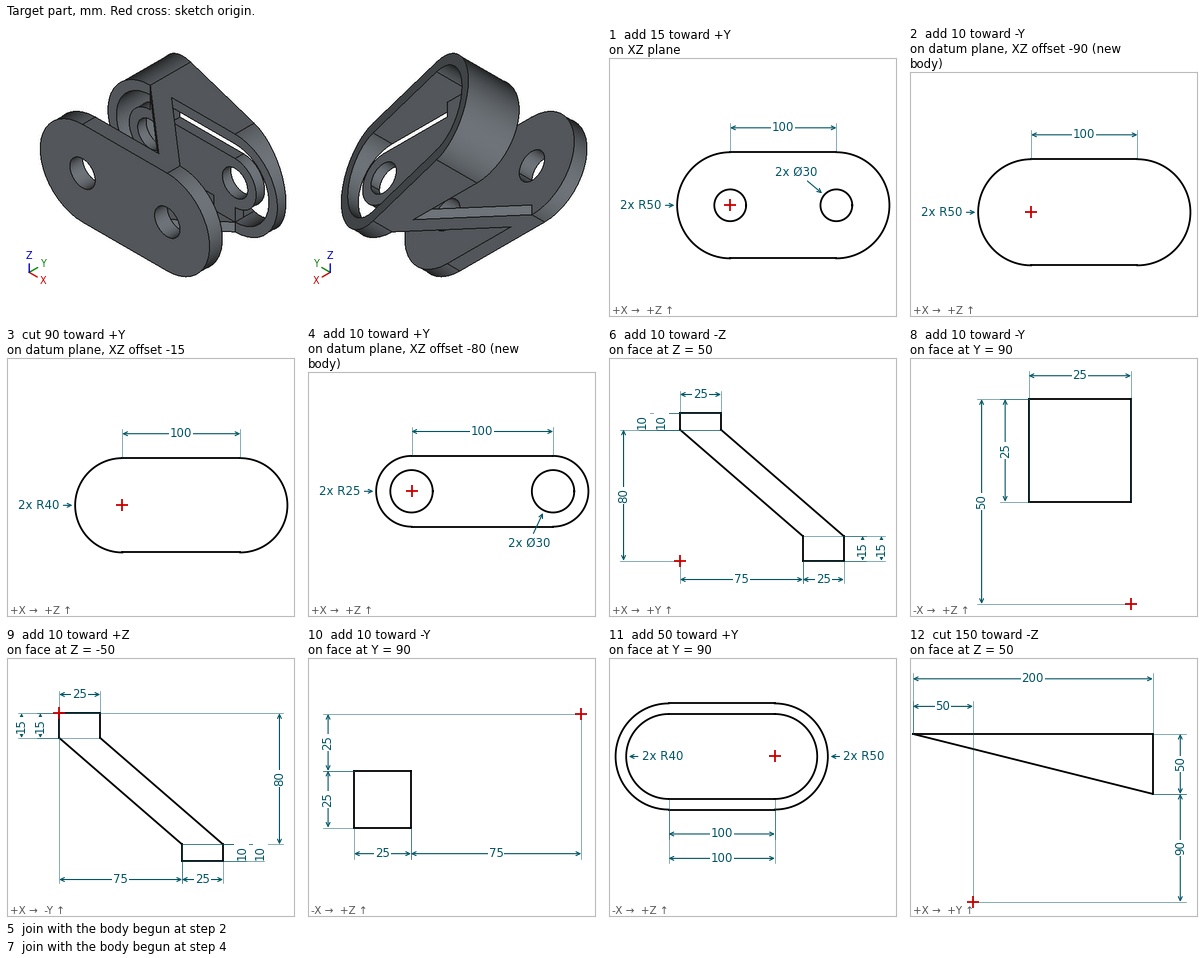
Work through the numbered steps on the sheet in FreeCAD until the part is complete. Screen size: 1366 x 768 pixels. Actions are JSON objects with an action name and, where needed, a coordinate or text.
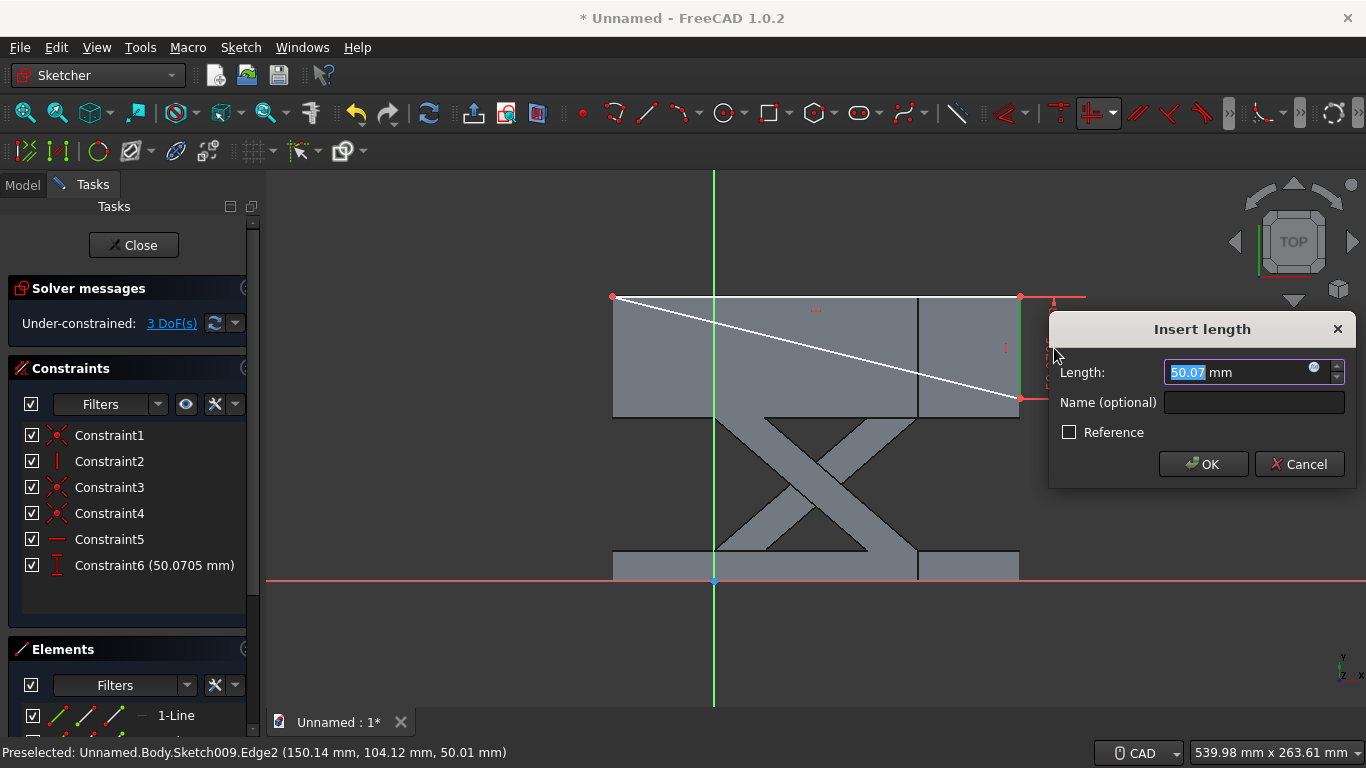
{"action": "type", "text": "50"}
{"action": "key", "text": "Return"}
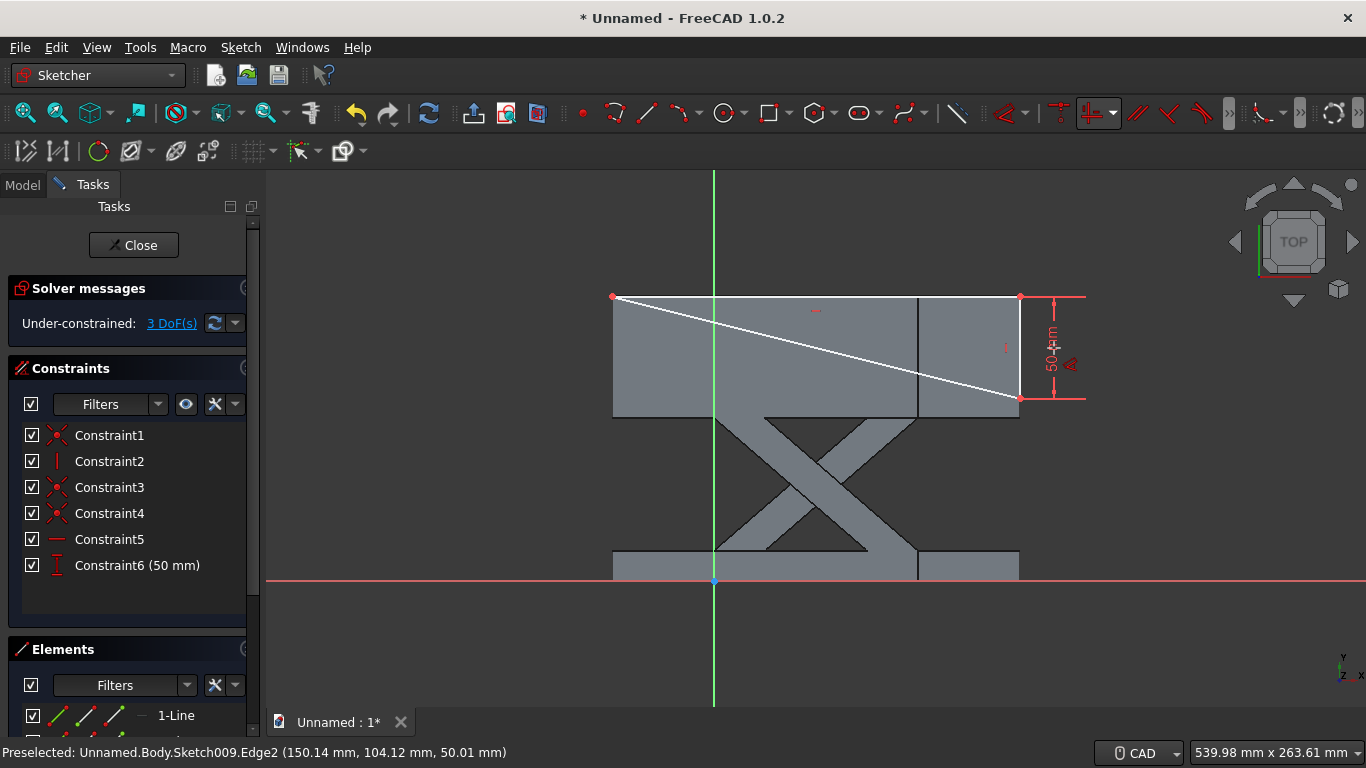
{"action": "left_click", "coordinate": [898, 297]}
{"action": "left_click", "coordinate": [816, 263]}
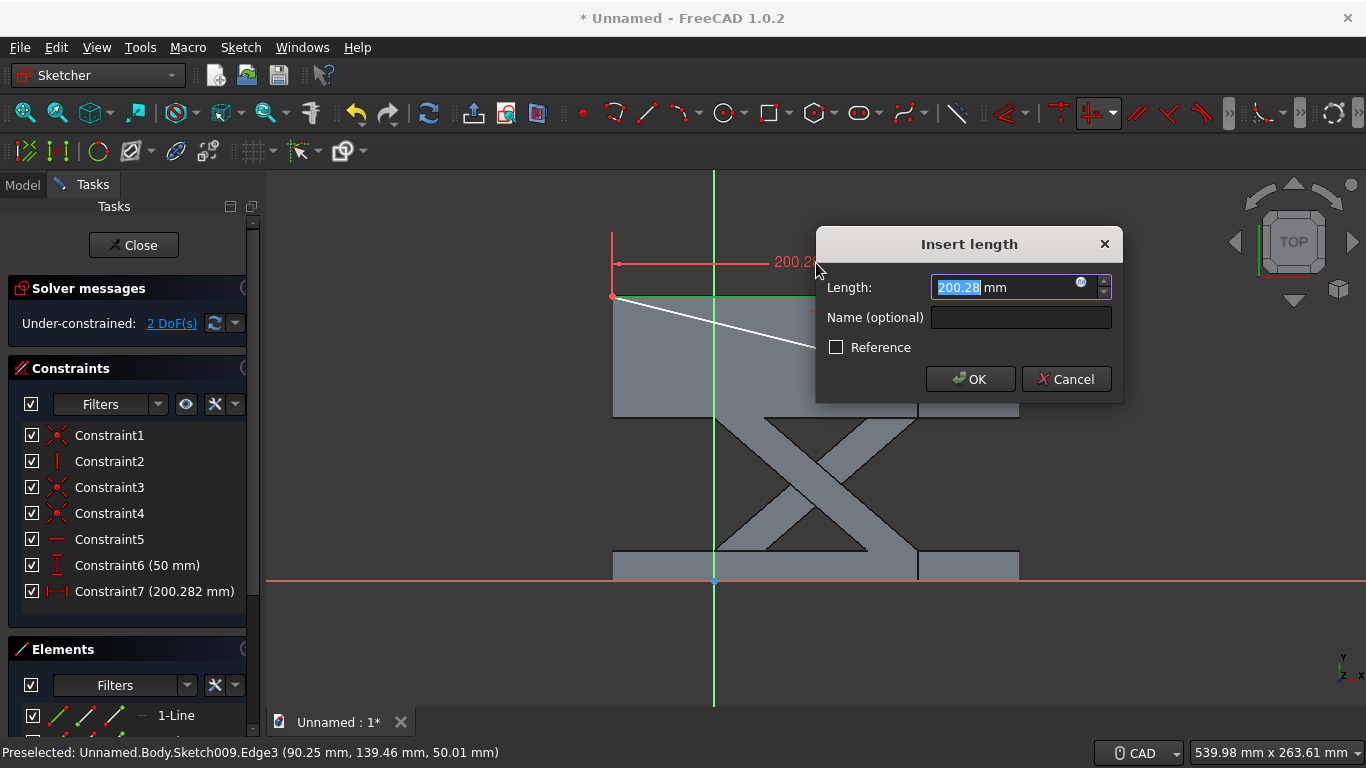
{"action": "type", "text": "200"}
{"action": "key", "text": "Return"}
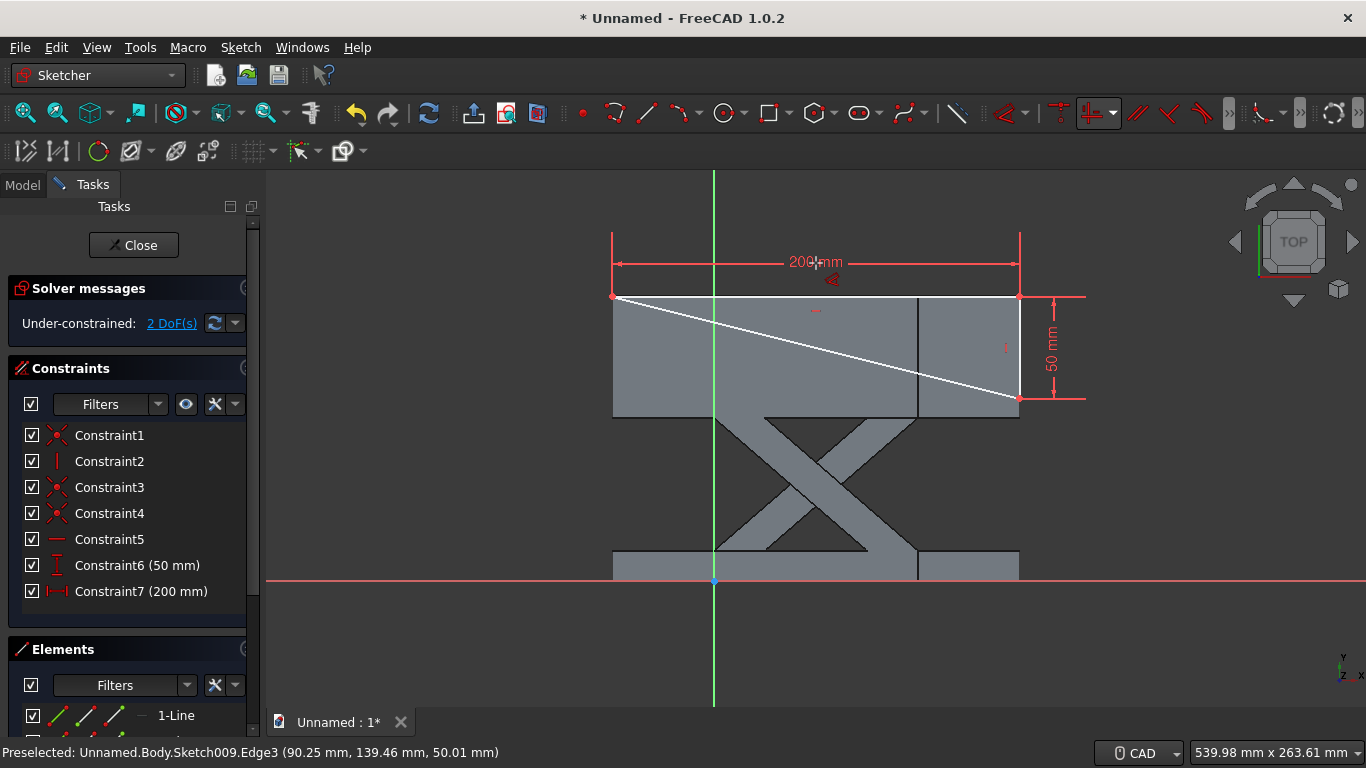
{"action": "left_click", "coordinate": [612, 297]}
{"action": "left_click", "coordinate": [663, 615]}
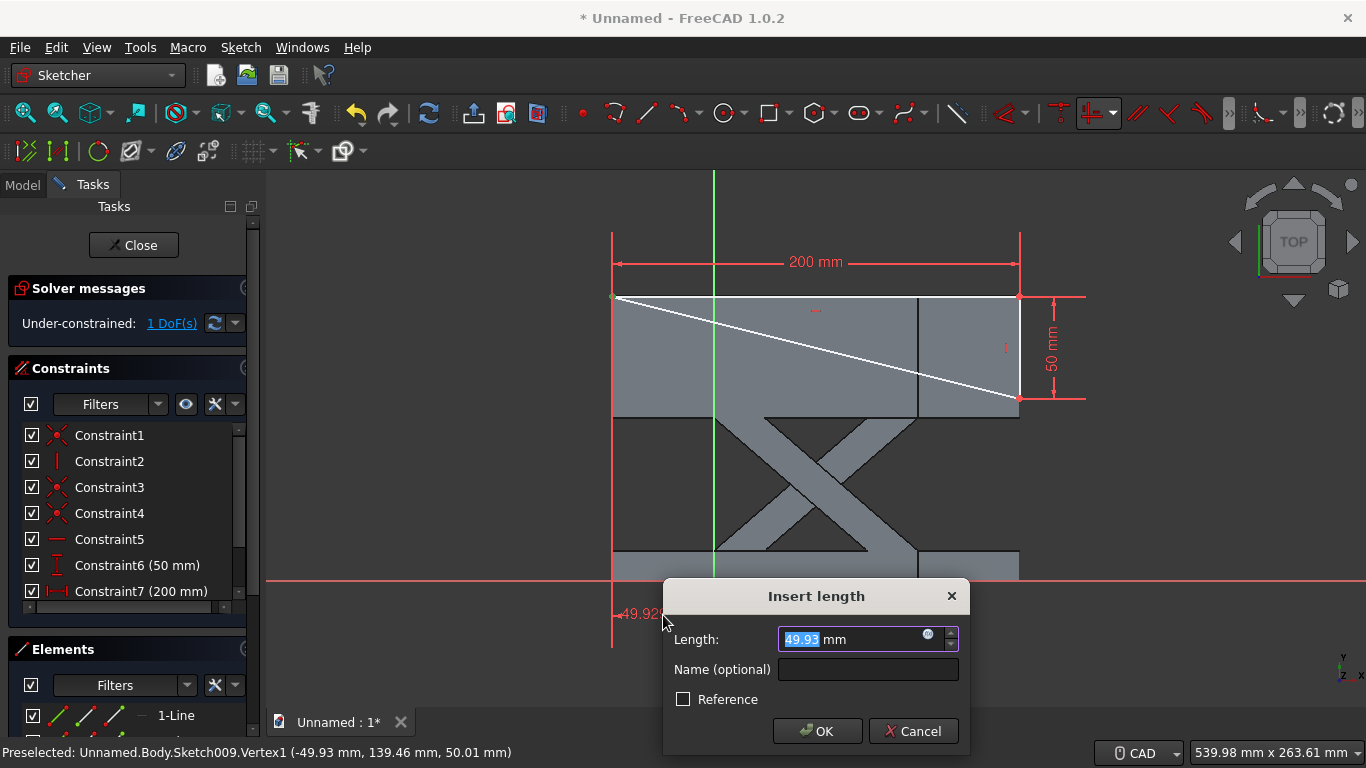
{"action": "type", "text": "50"}
{"action": "key", "text": "Return"}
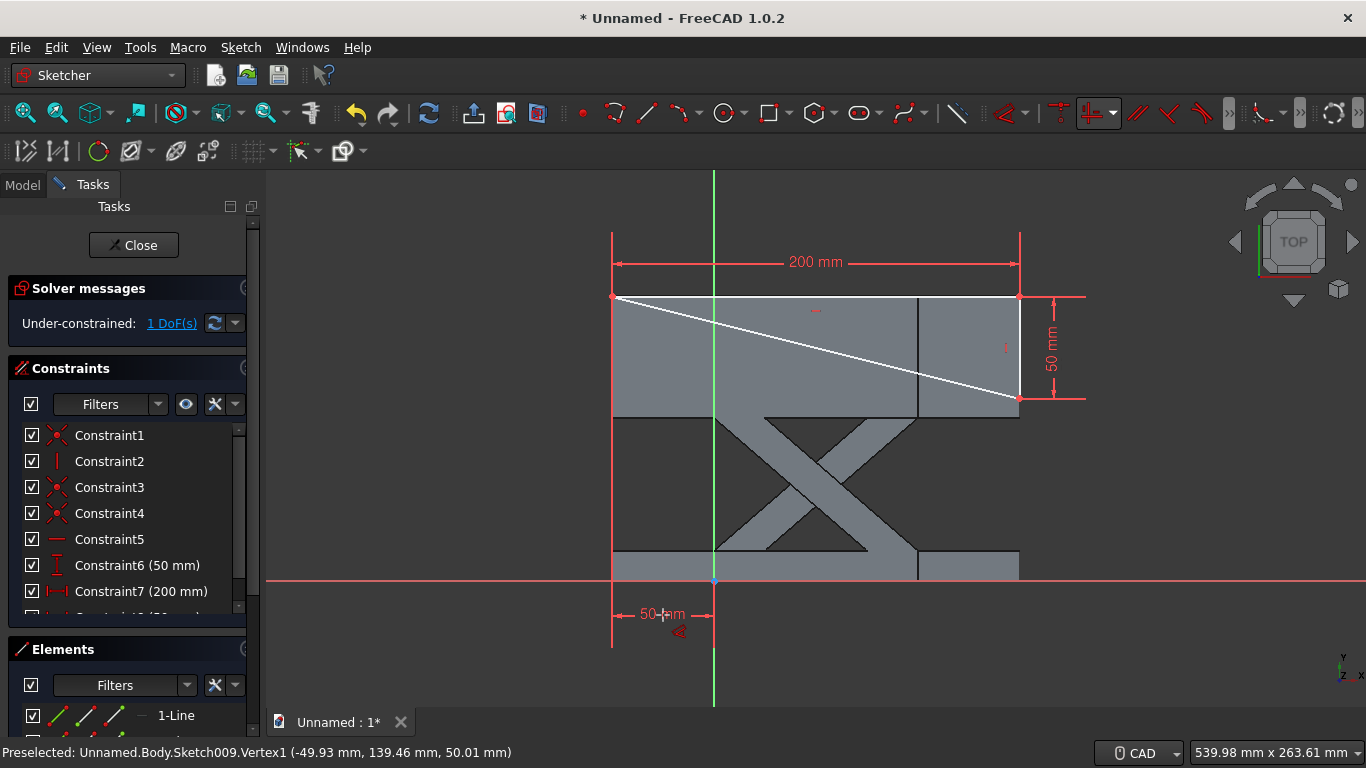
{"action": "left_click", "coordinate": [1020, 399]}
{"action": "left_click", "coordinate": [1054, 490]}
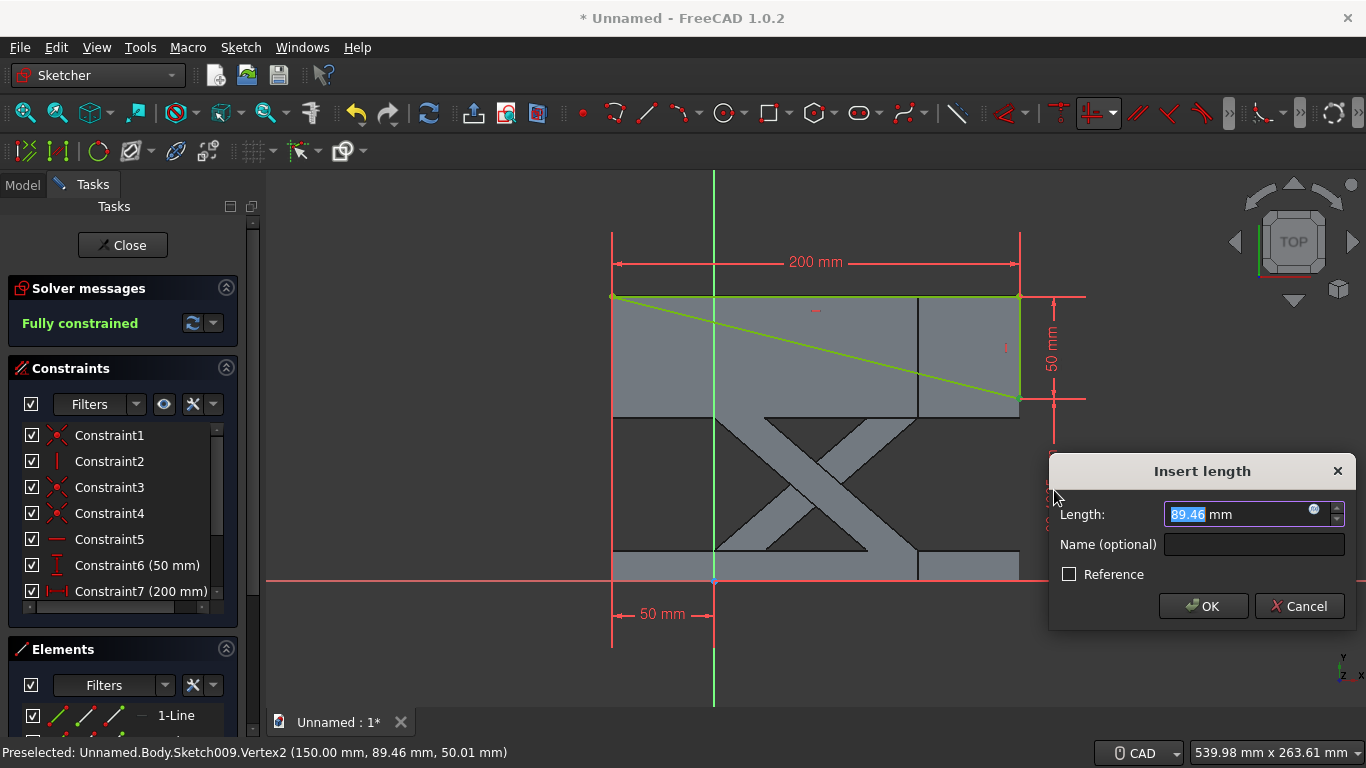
{"action": "type", "text": "90"}
{"action": "key", "text": "Return"}
{"action": "key", "text": "Escape"}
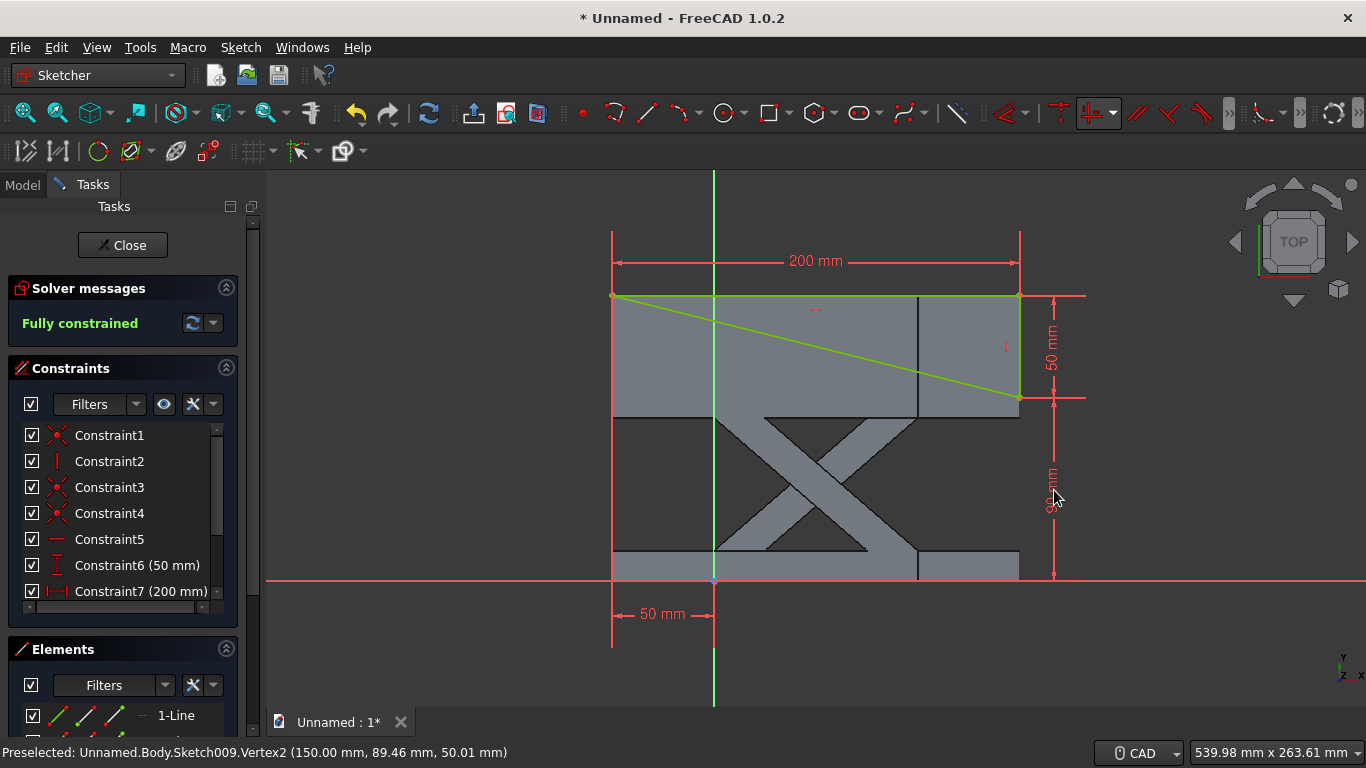
{"action": "left_click", "coordinate": [123, 245]}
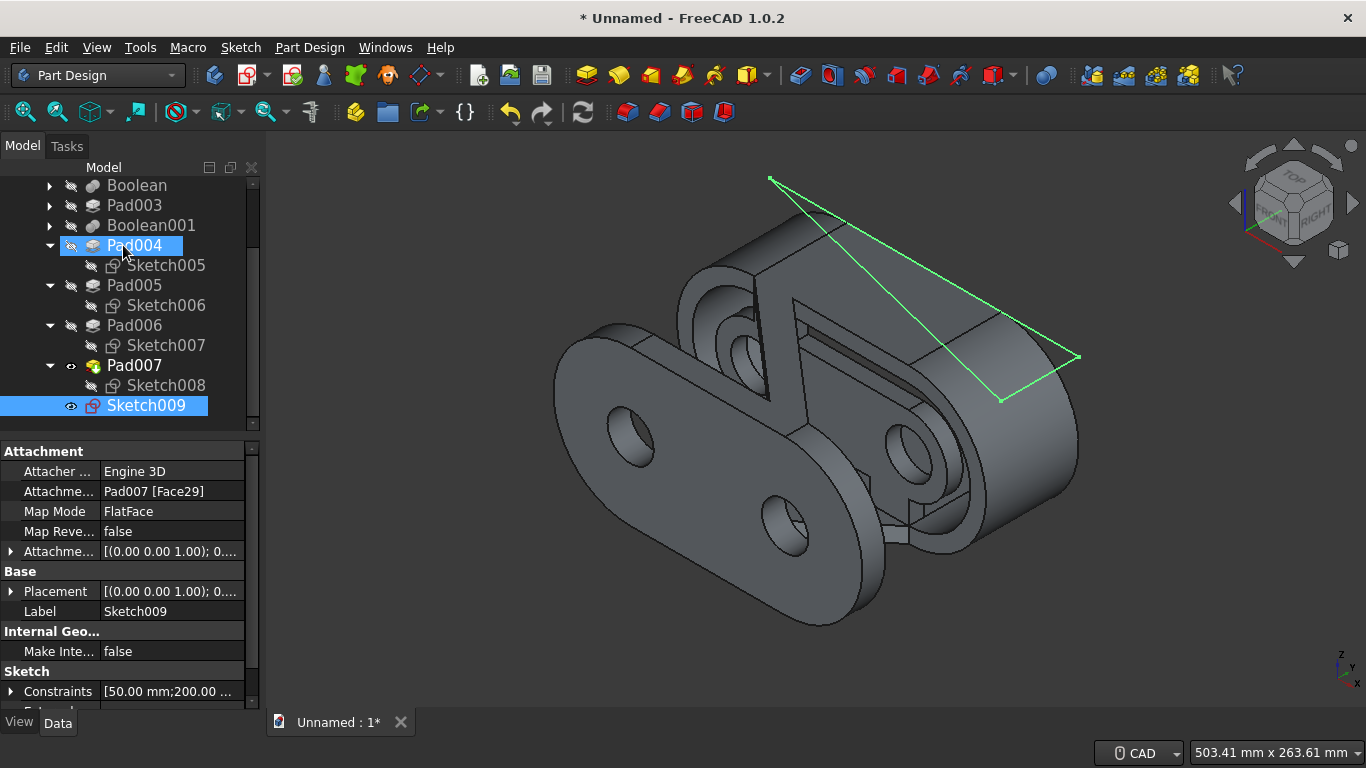
{"action": "left_click", "coordinate": [802, 76]}